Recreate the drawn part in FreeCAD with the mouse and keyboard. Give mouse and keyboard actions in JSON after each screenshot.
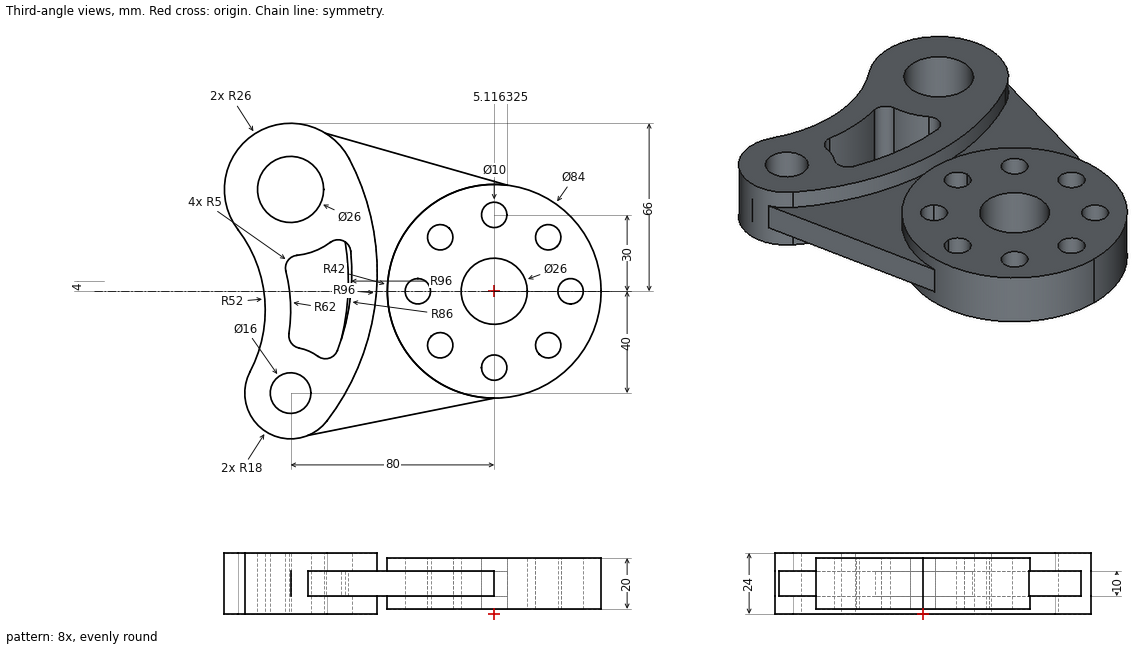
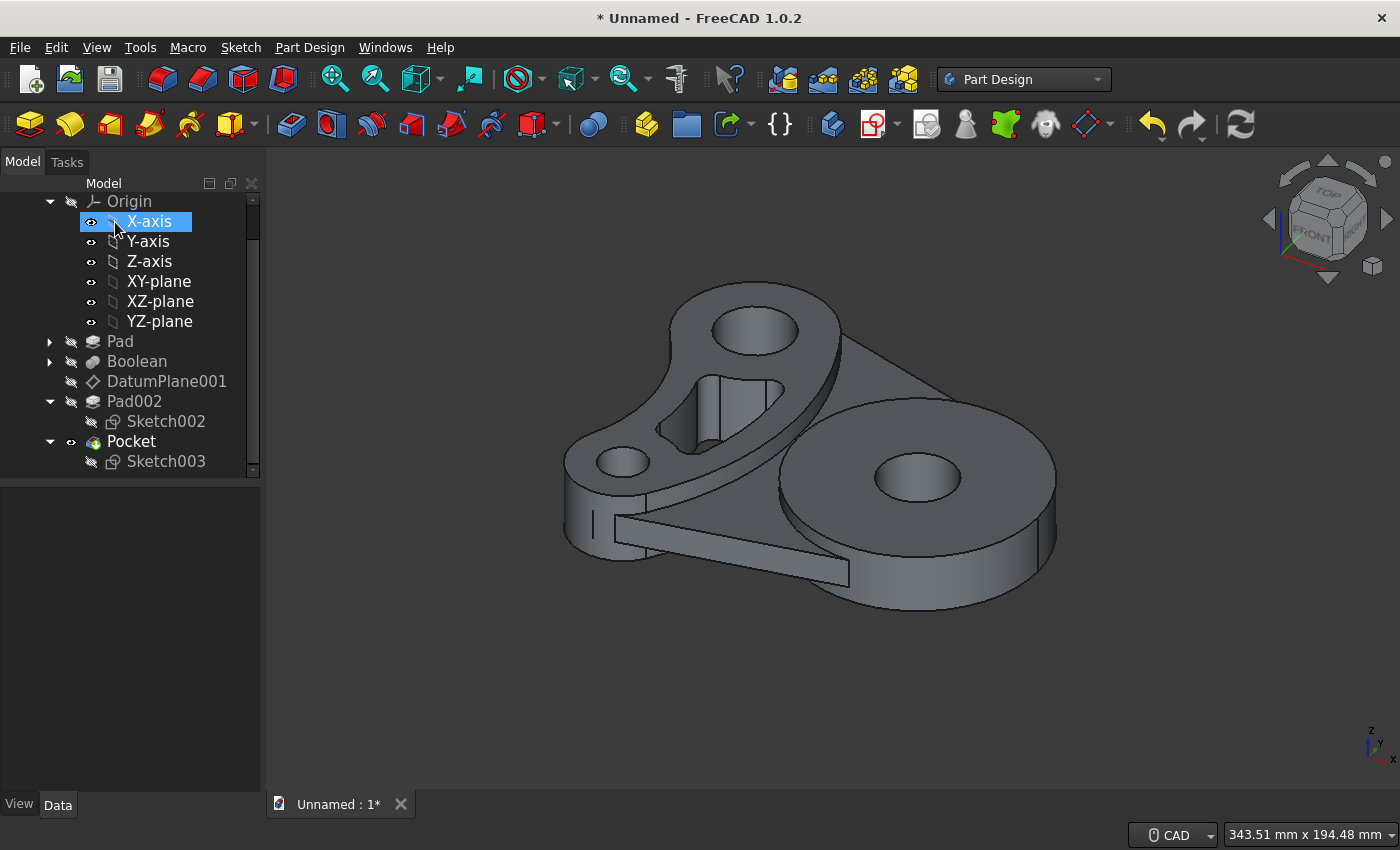
{"action": "left_click", "coordinate": [869, 434]}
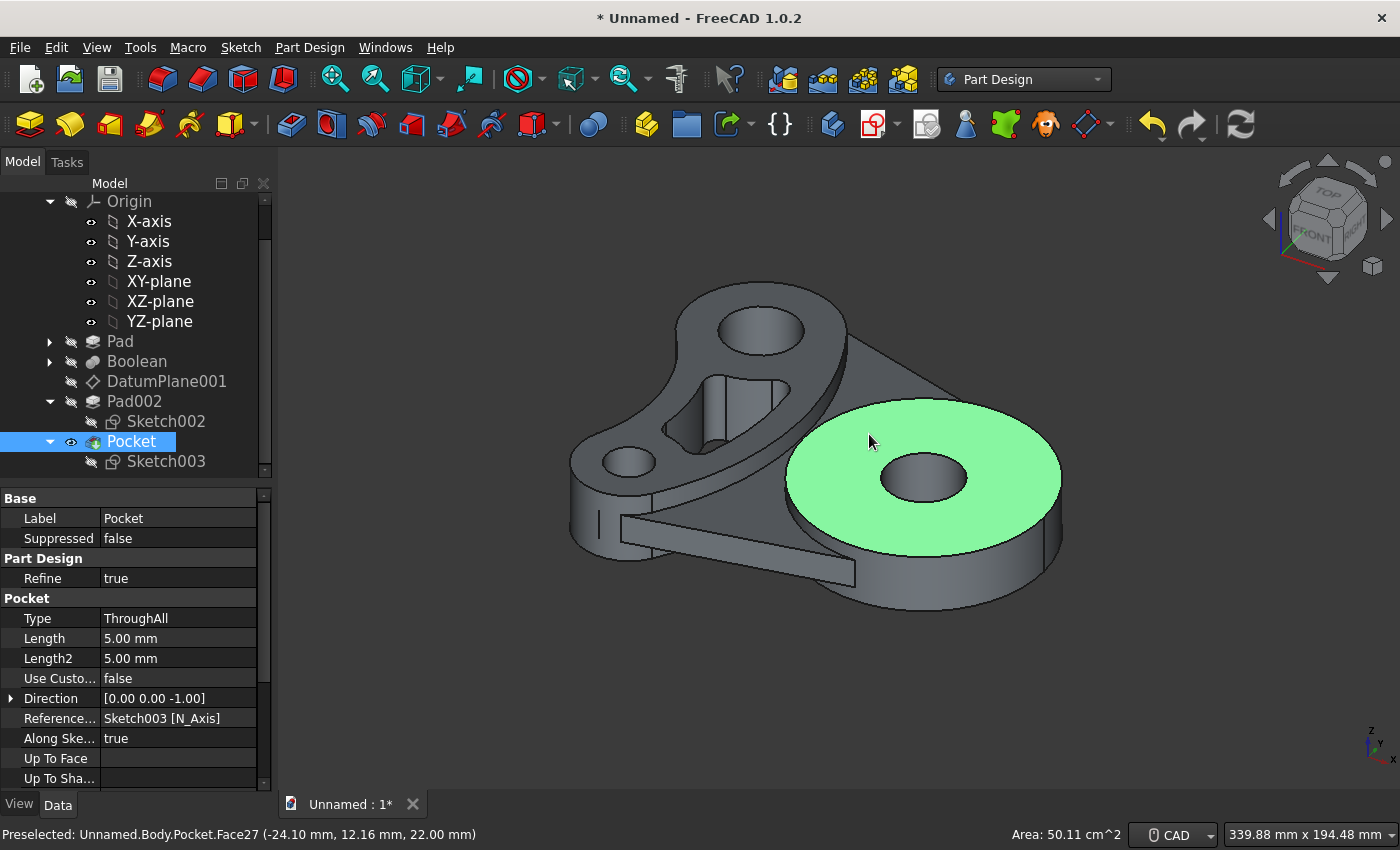
{"action": "left_click", "coordinate": [874, 124]}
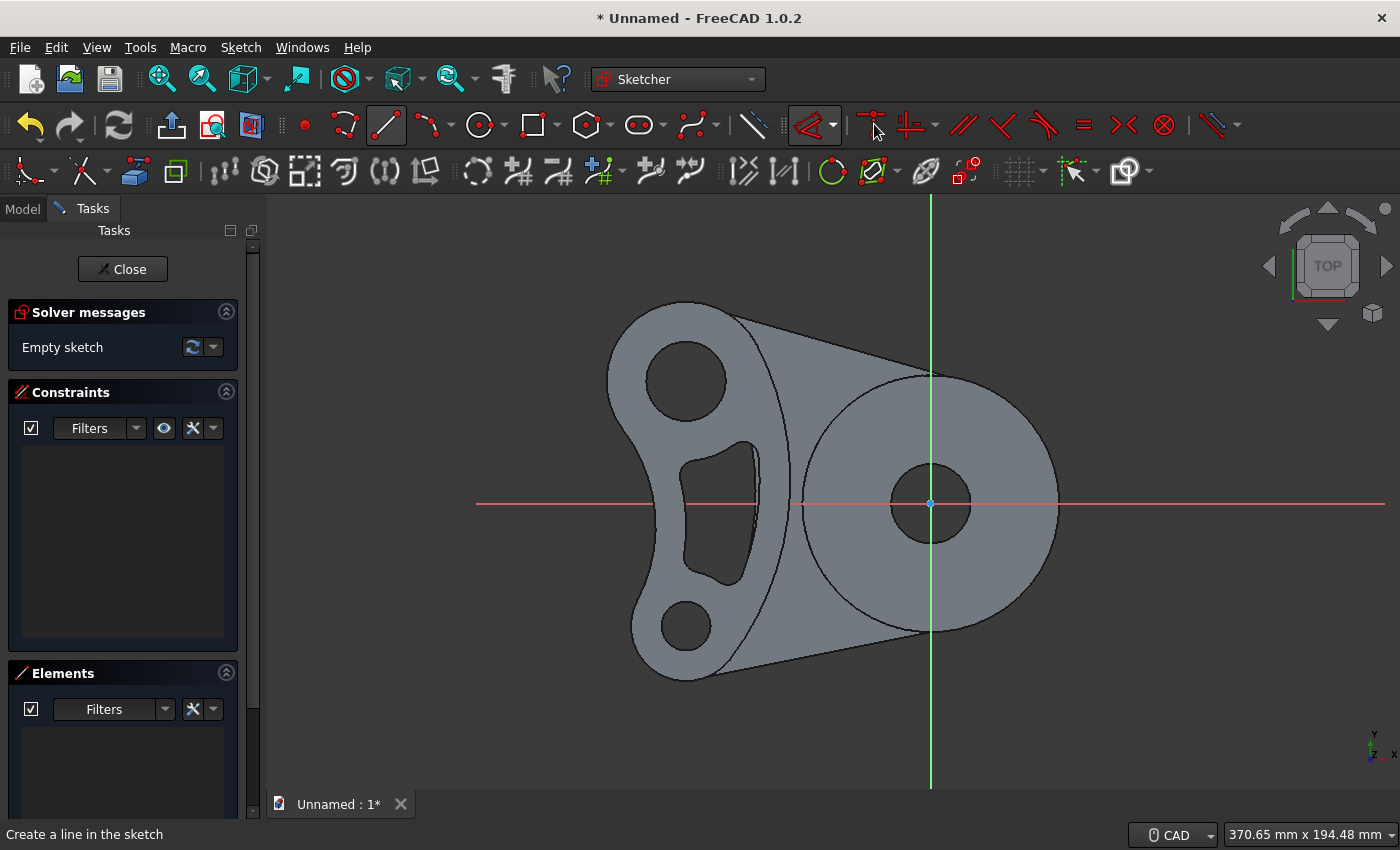
{"action": "left_click", "coordinate": [252, 126]}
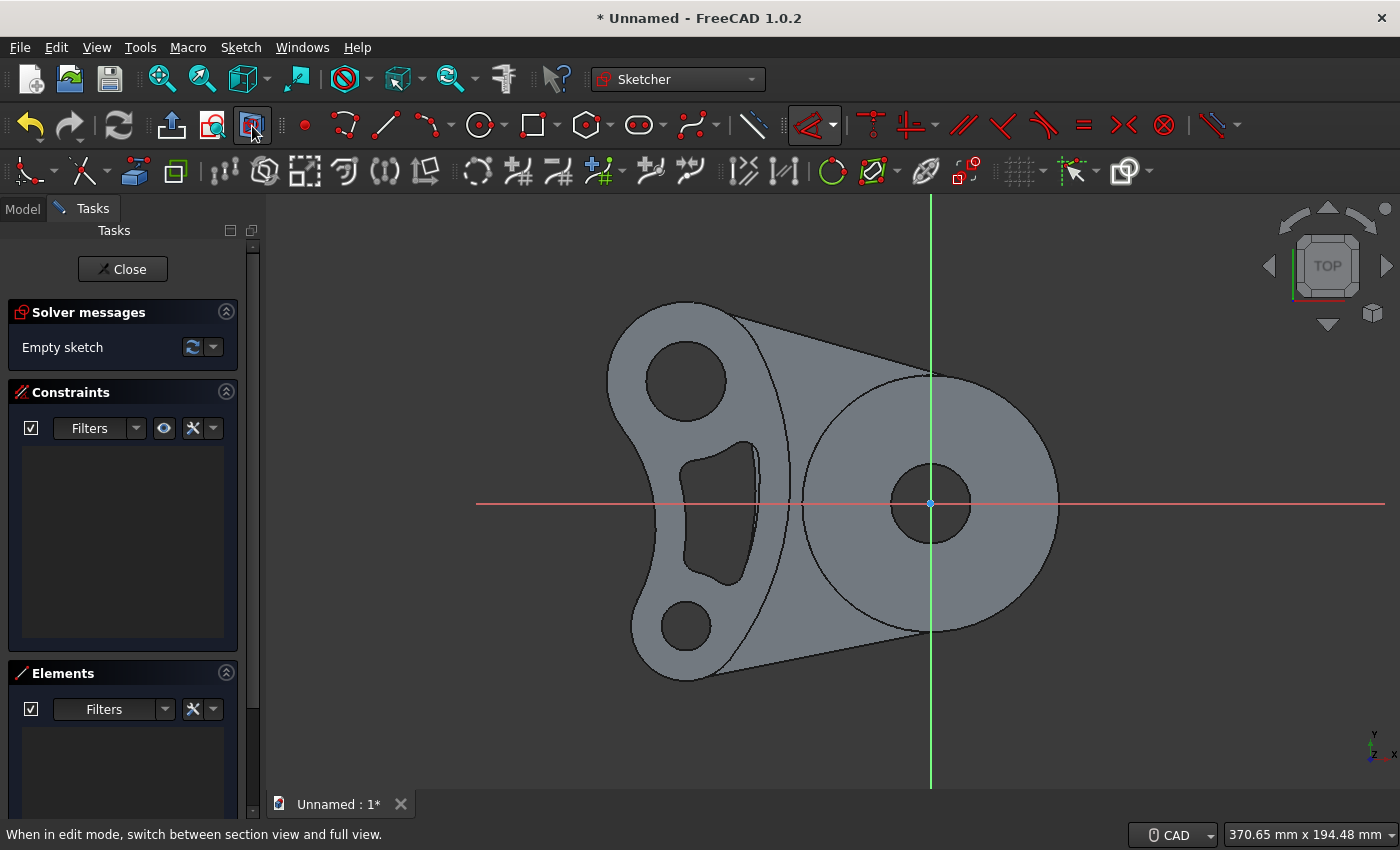
{"action": "scroll", "coordinate": [944, 406], "scroll_direction": "up", "scroll_amount": 13}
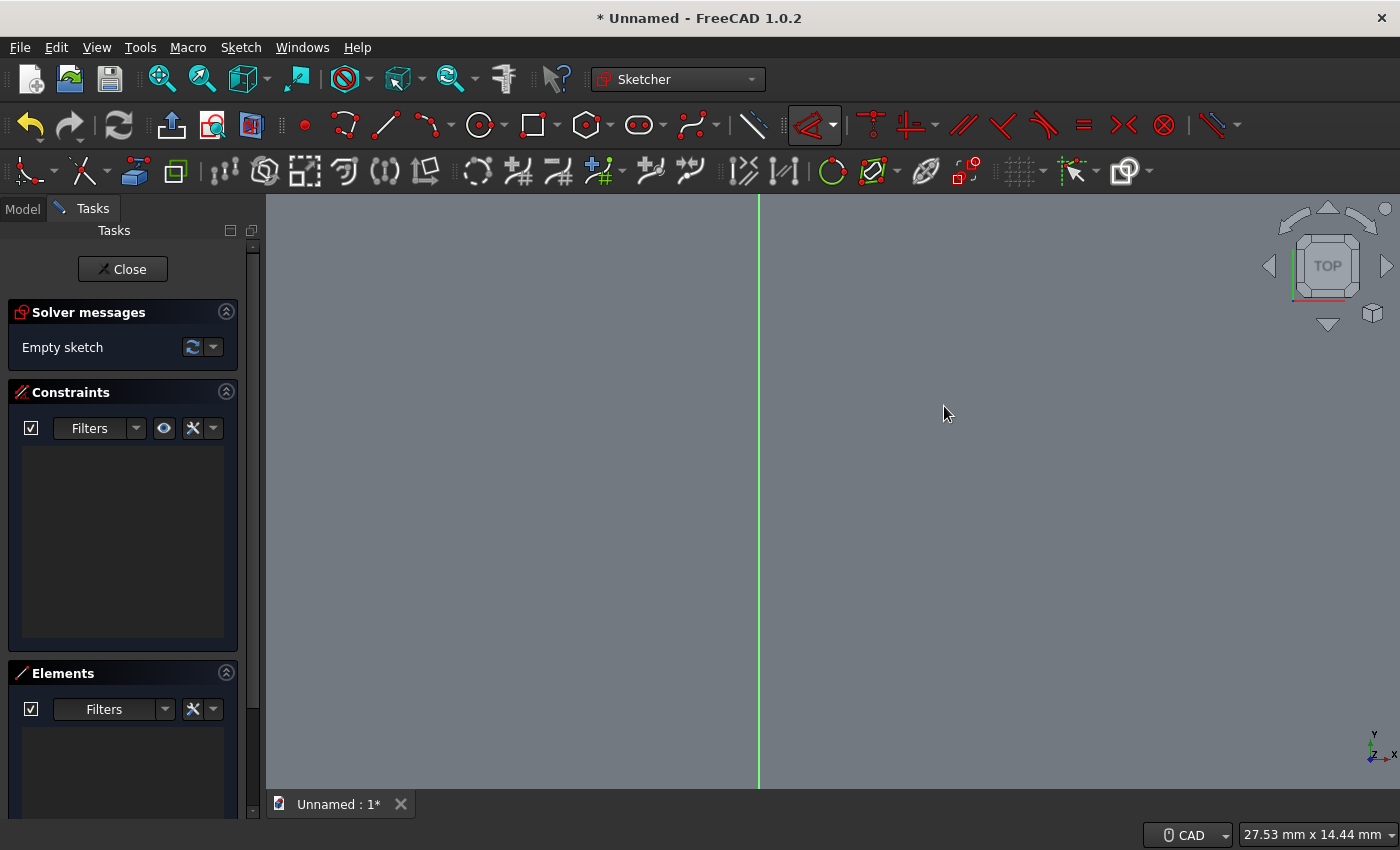
{"action": "left_click", "coordinate": [480, 126]}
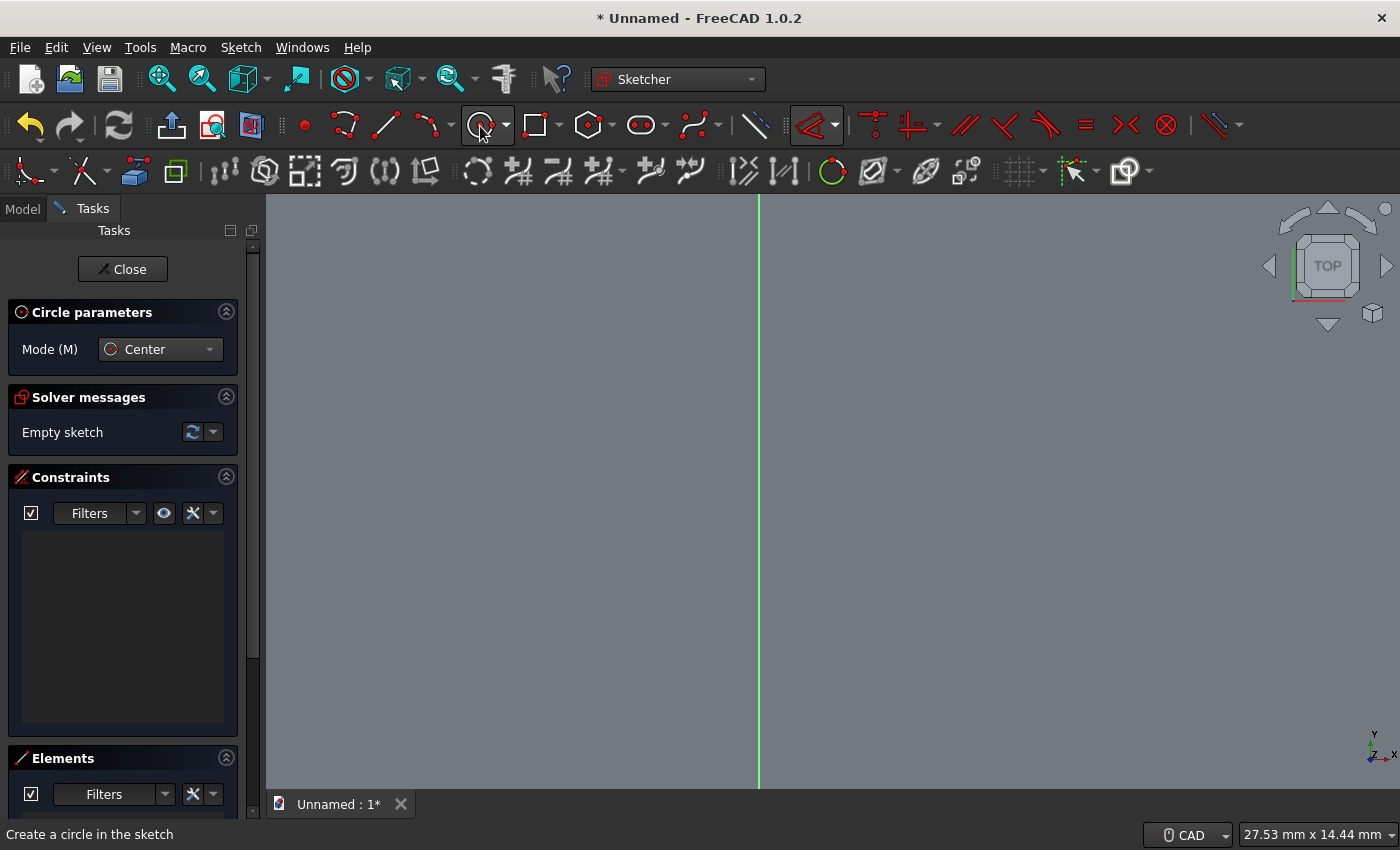
{"action": "left_click", "coordinate": [759, 481]}
{"action": "left_click", "coordinate": [905, 336]}
{"action": "key", "text": "Escape"}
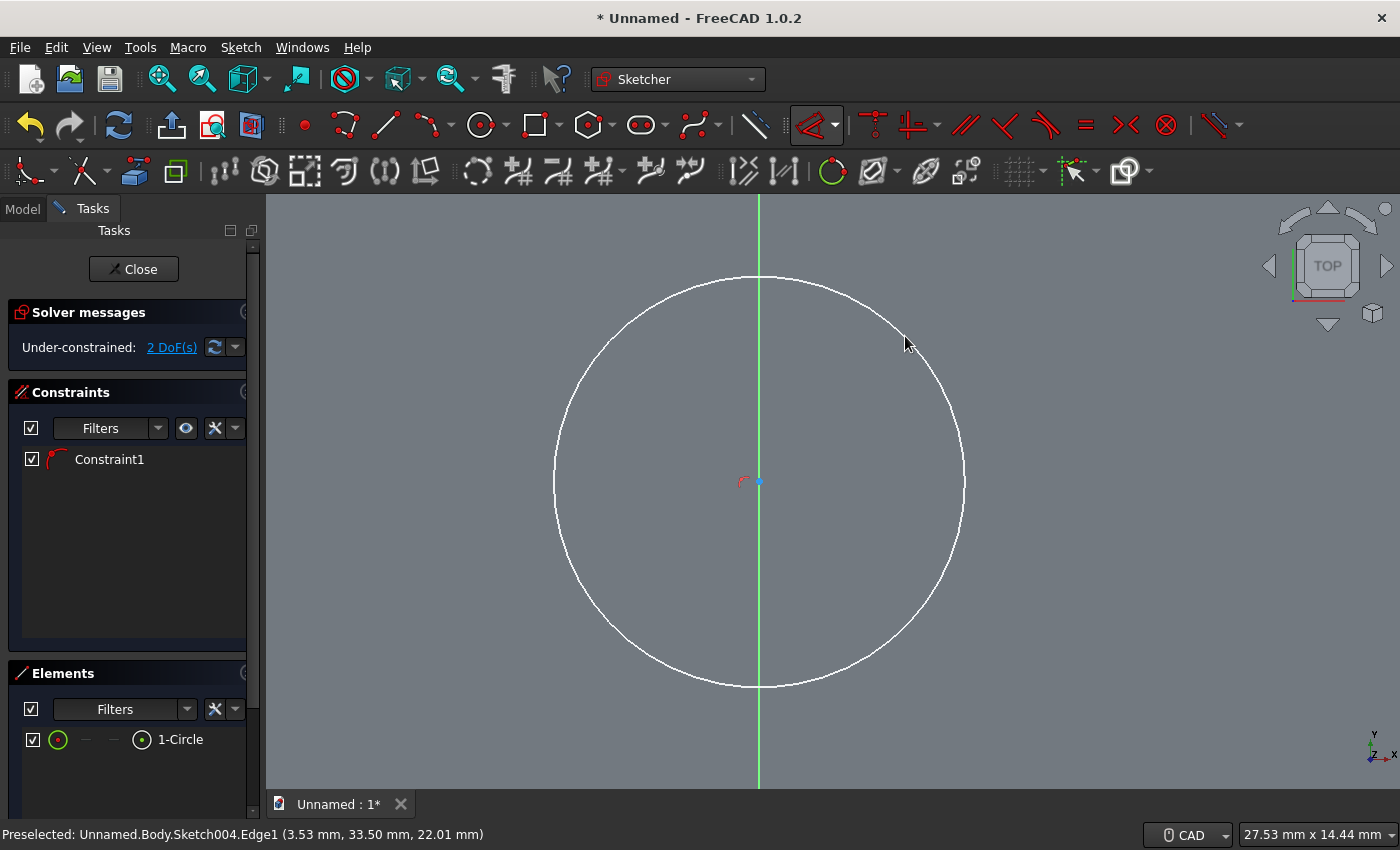
{"action": "left_click", "coordinate": [904, 336]}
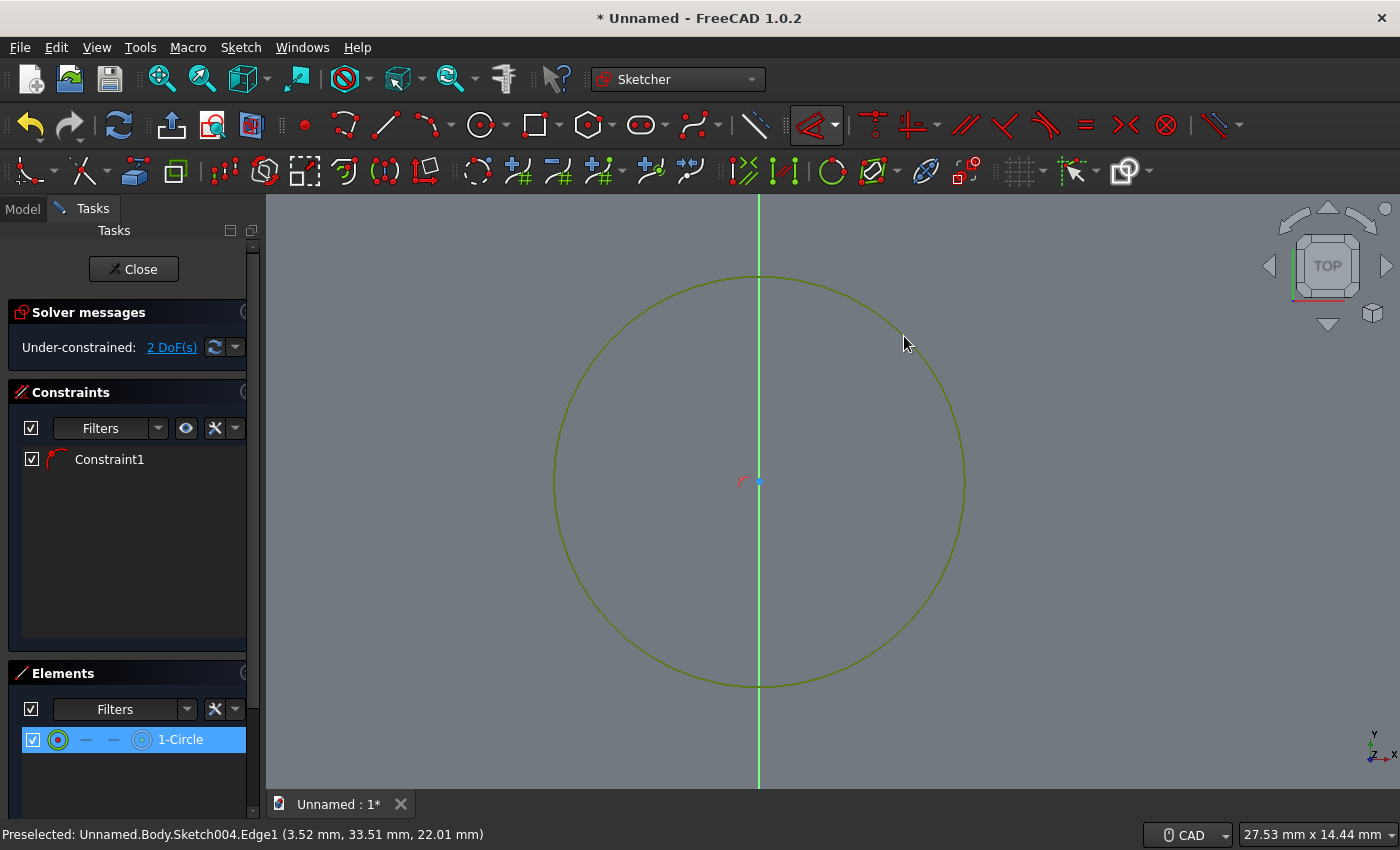
{"action": "left_click", "coordinate": [838, 126]}